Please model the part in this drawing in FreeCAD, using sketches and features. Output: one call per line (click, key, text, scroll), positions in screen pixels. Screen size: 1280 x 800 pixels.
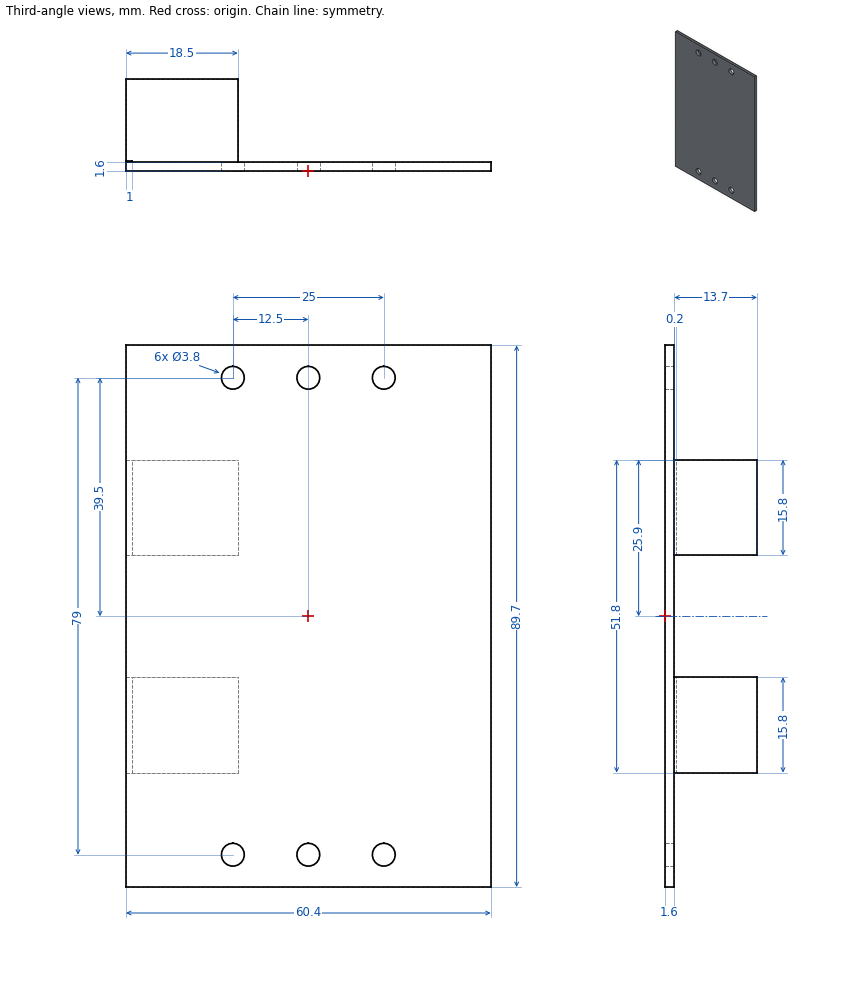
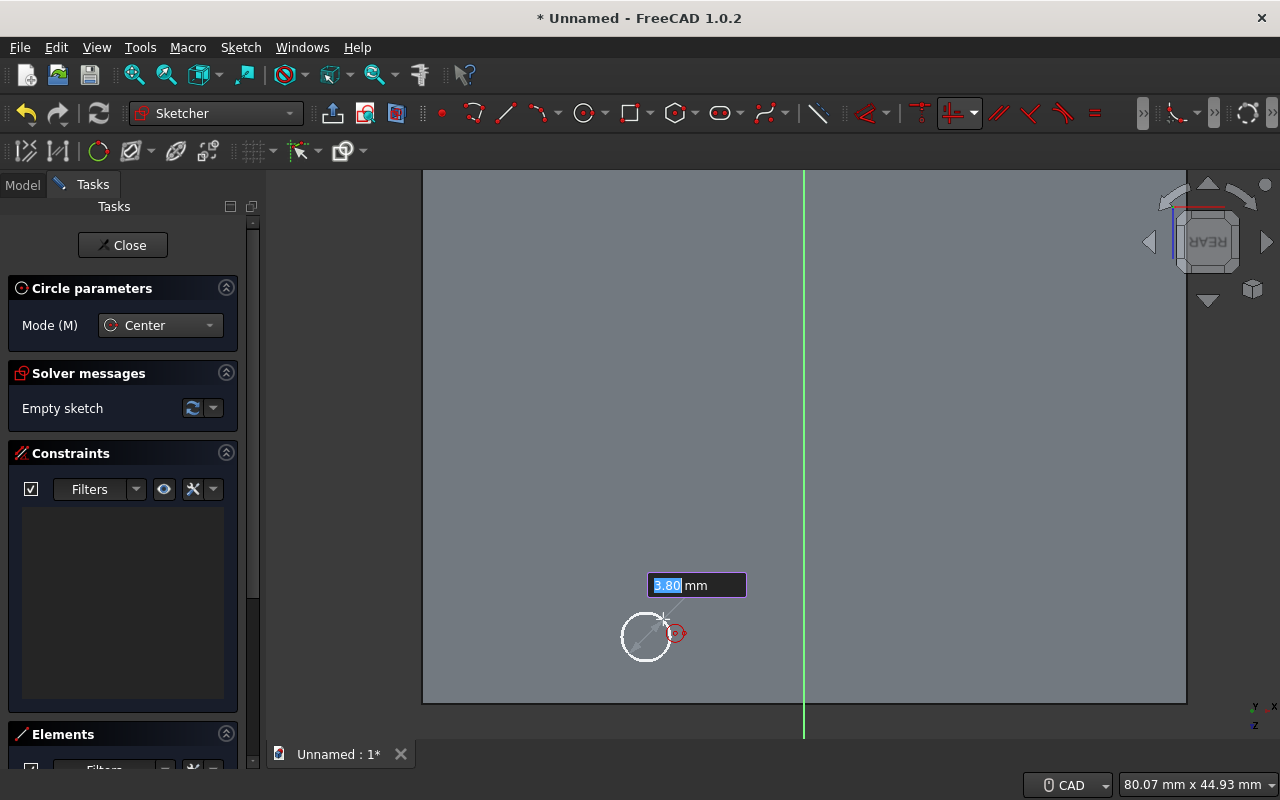
text(3.8)
key(Return)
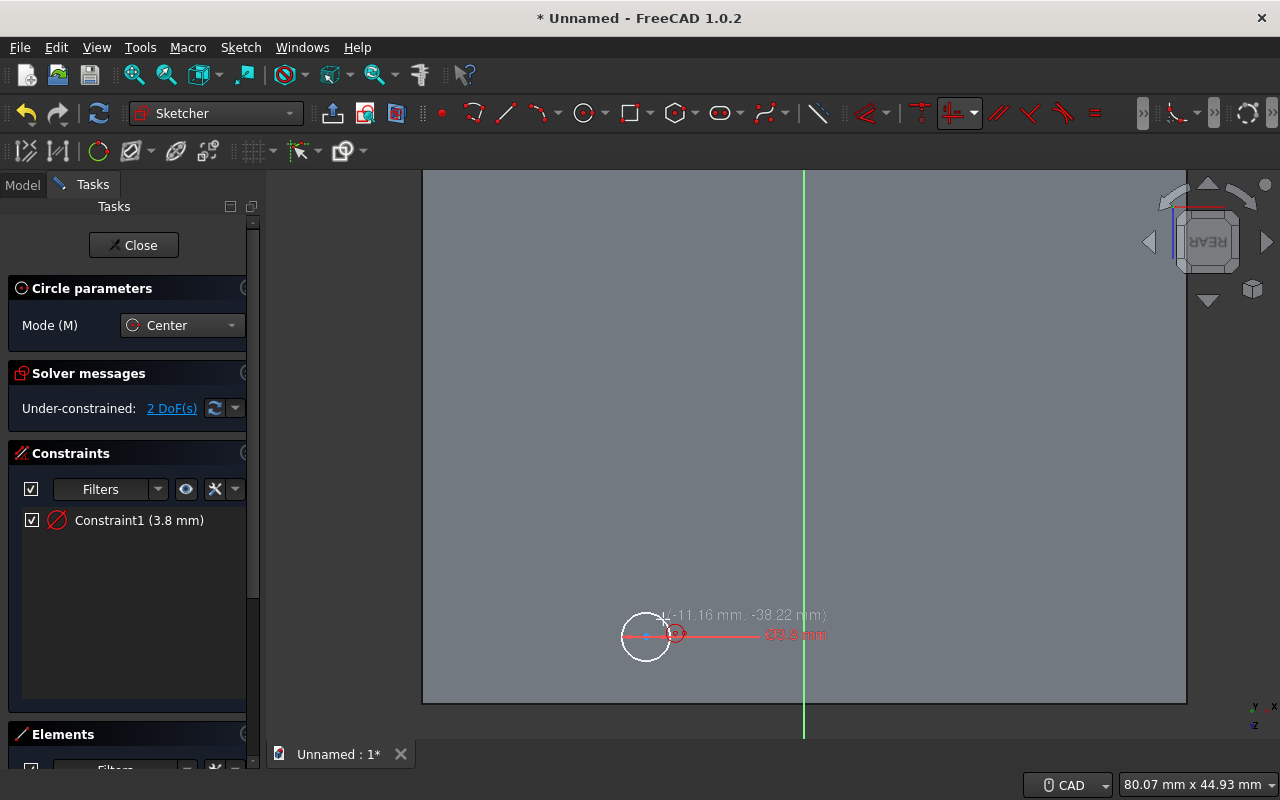
click(963, 636)
move(980, 619)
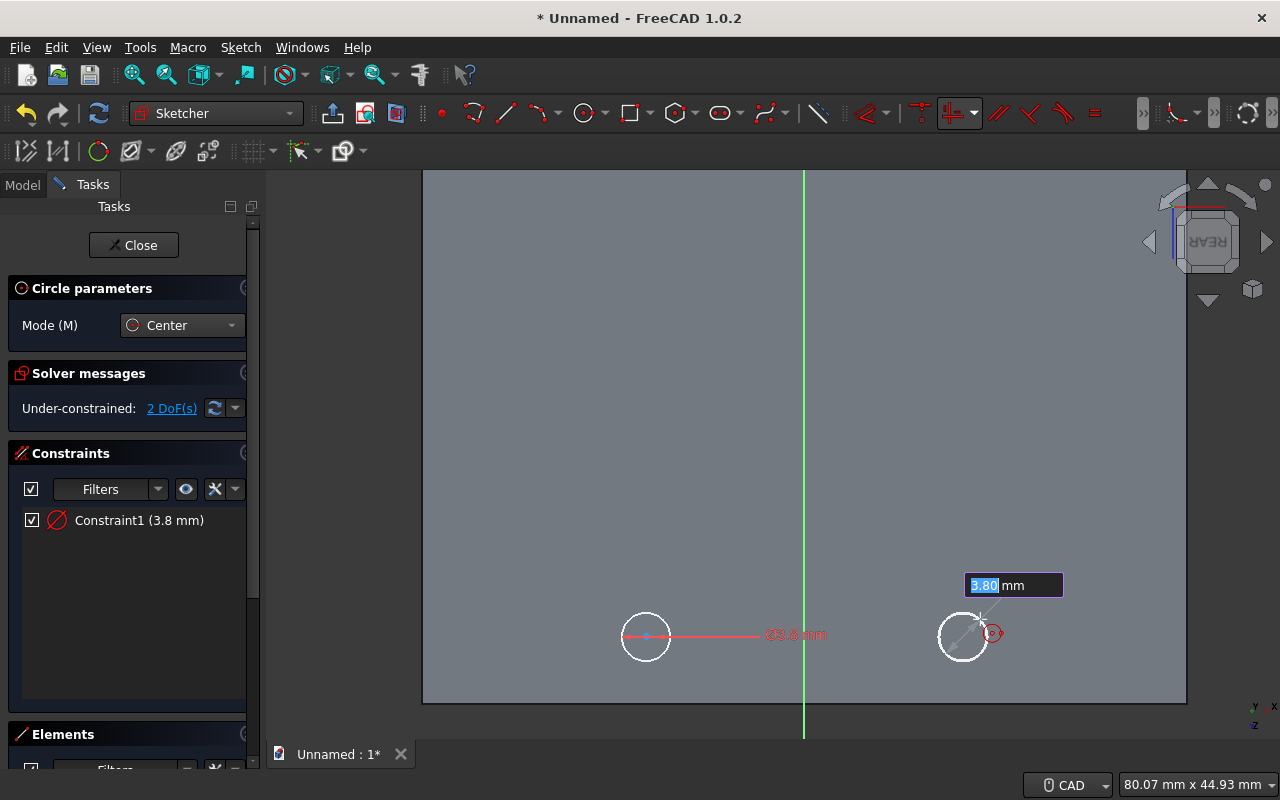
text(3.8)
key(Return)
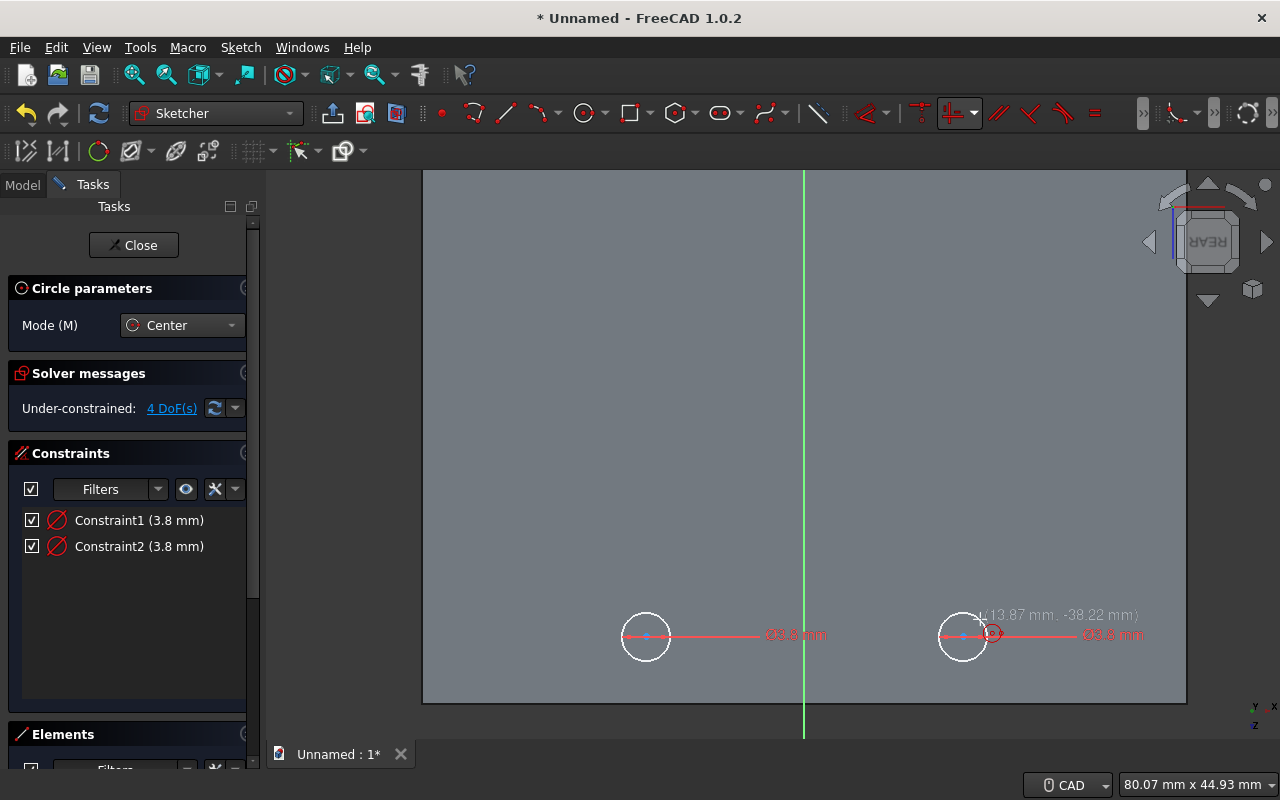
scroll(646, 640, down, 5)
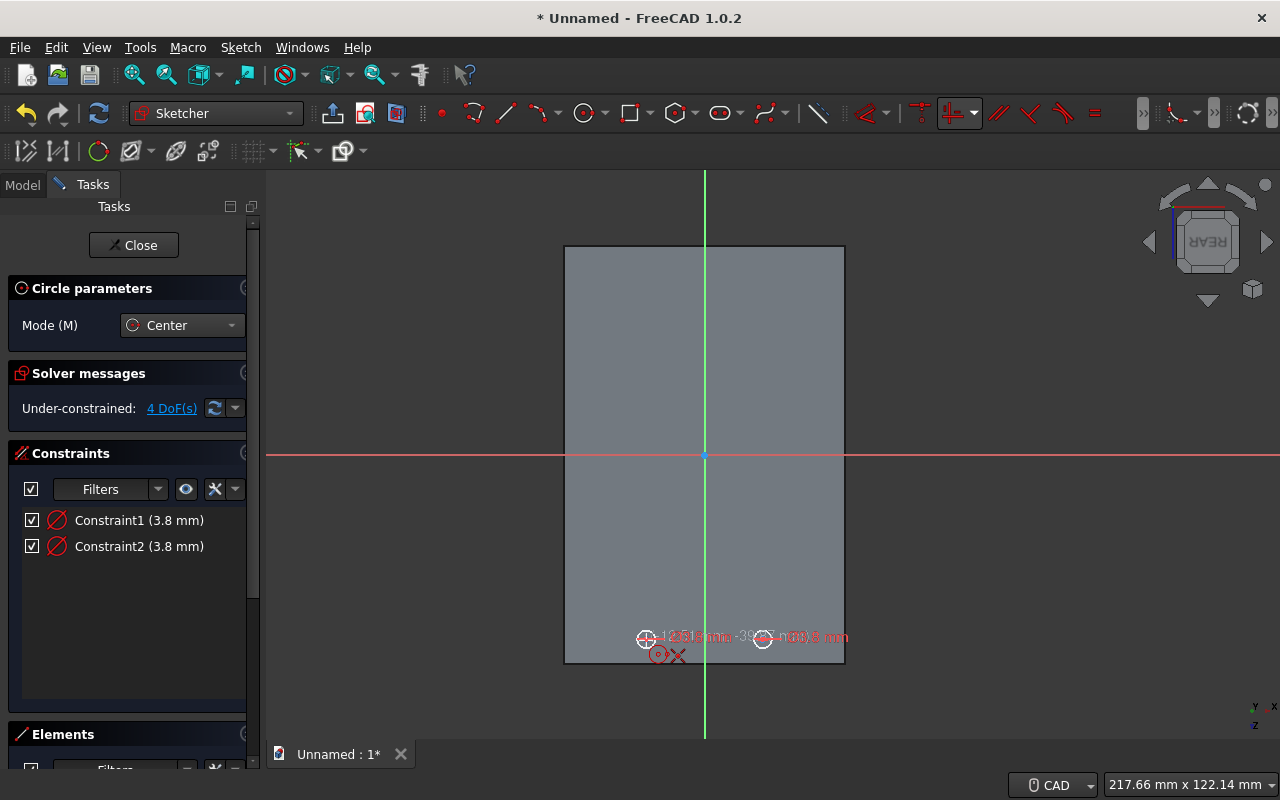
scroll(646, 271, up, 5)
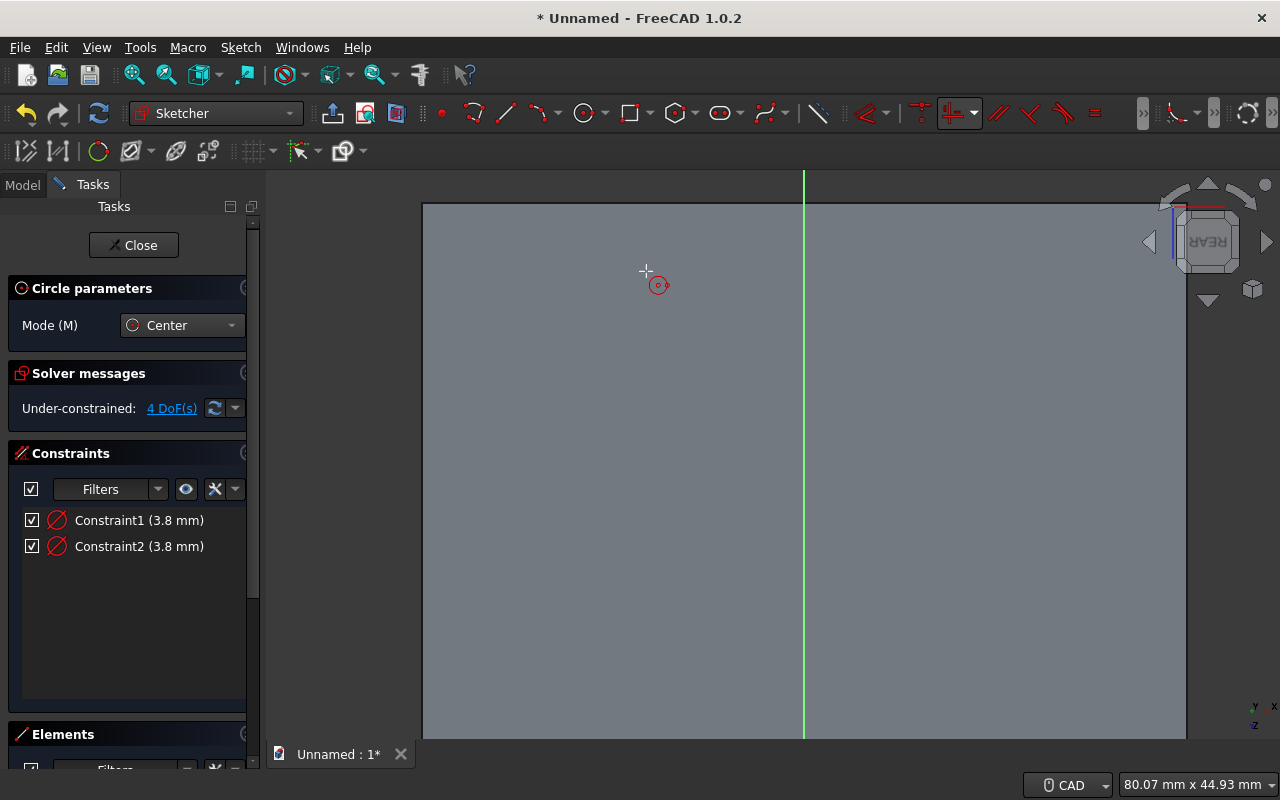
click(646, 271)
move(663, 254)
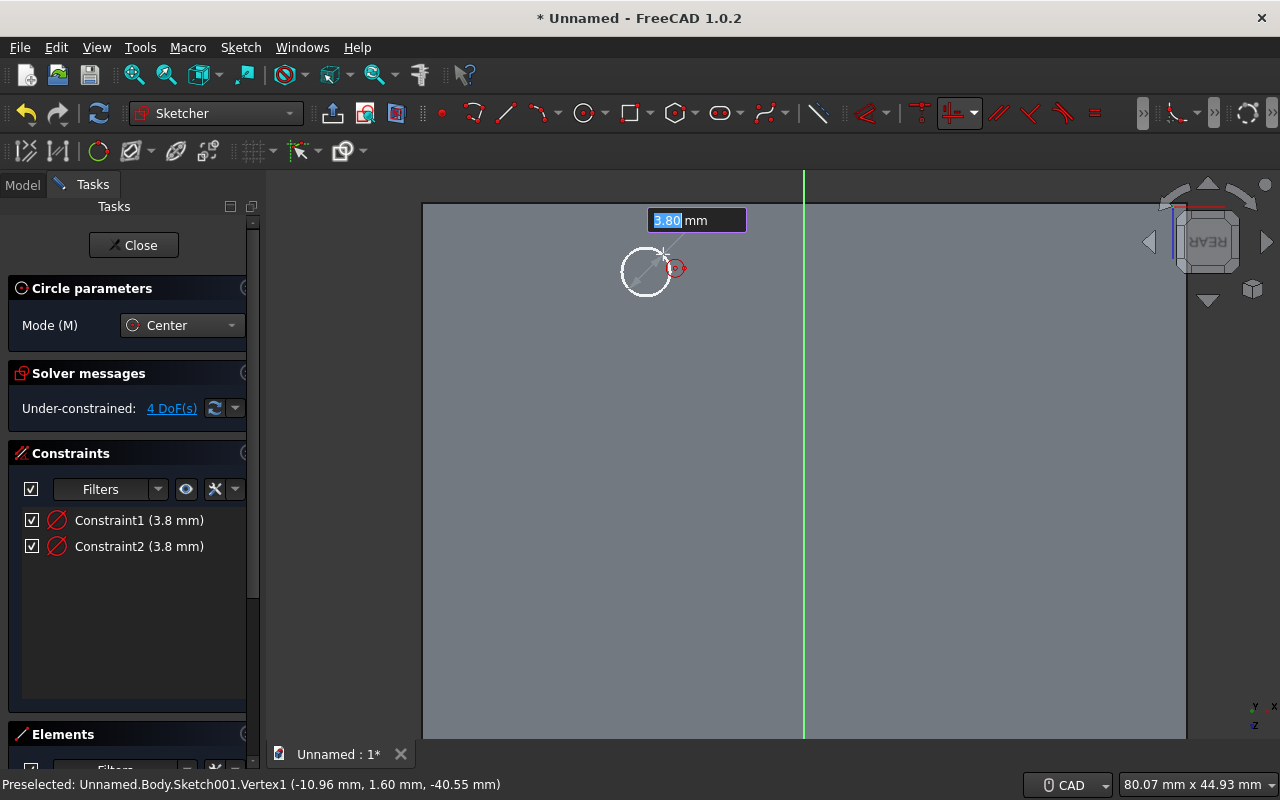
text(3.8)
key(Return)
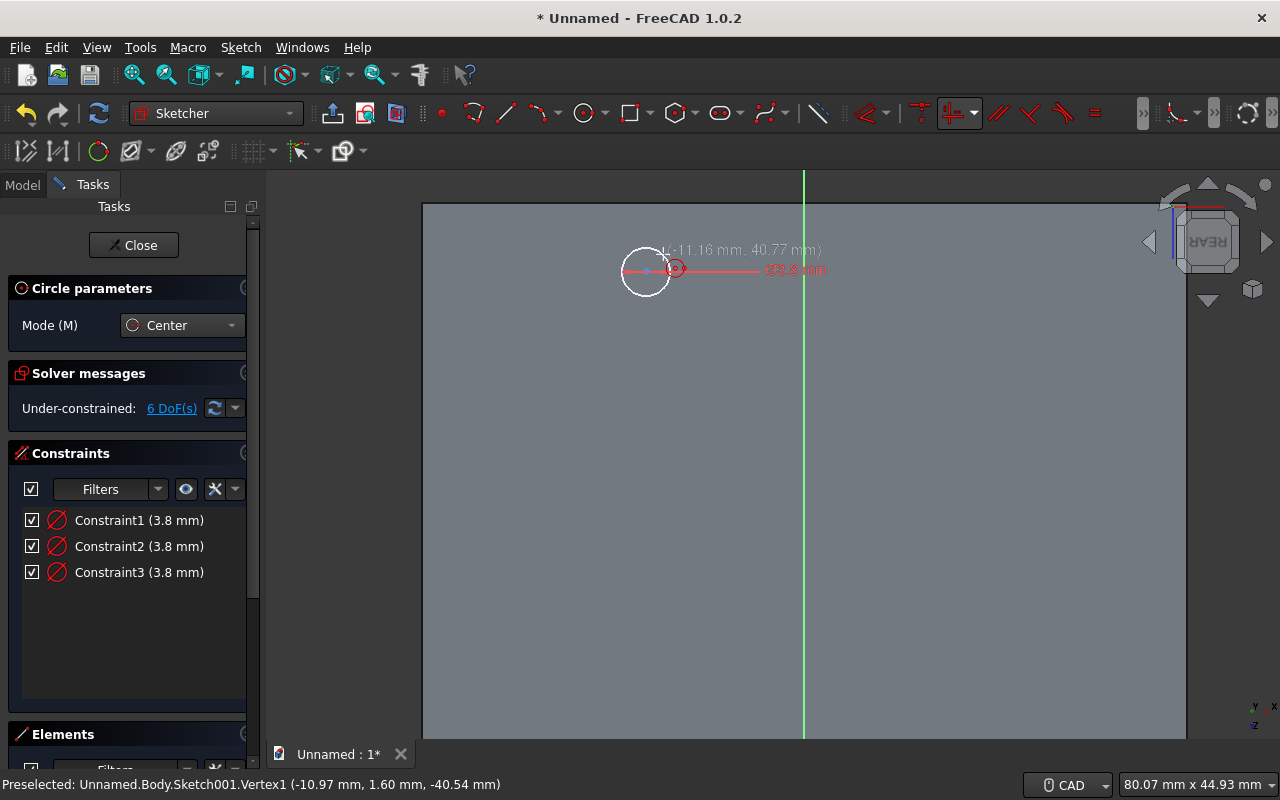
click(963, 271)
move(980, 254)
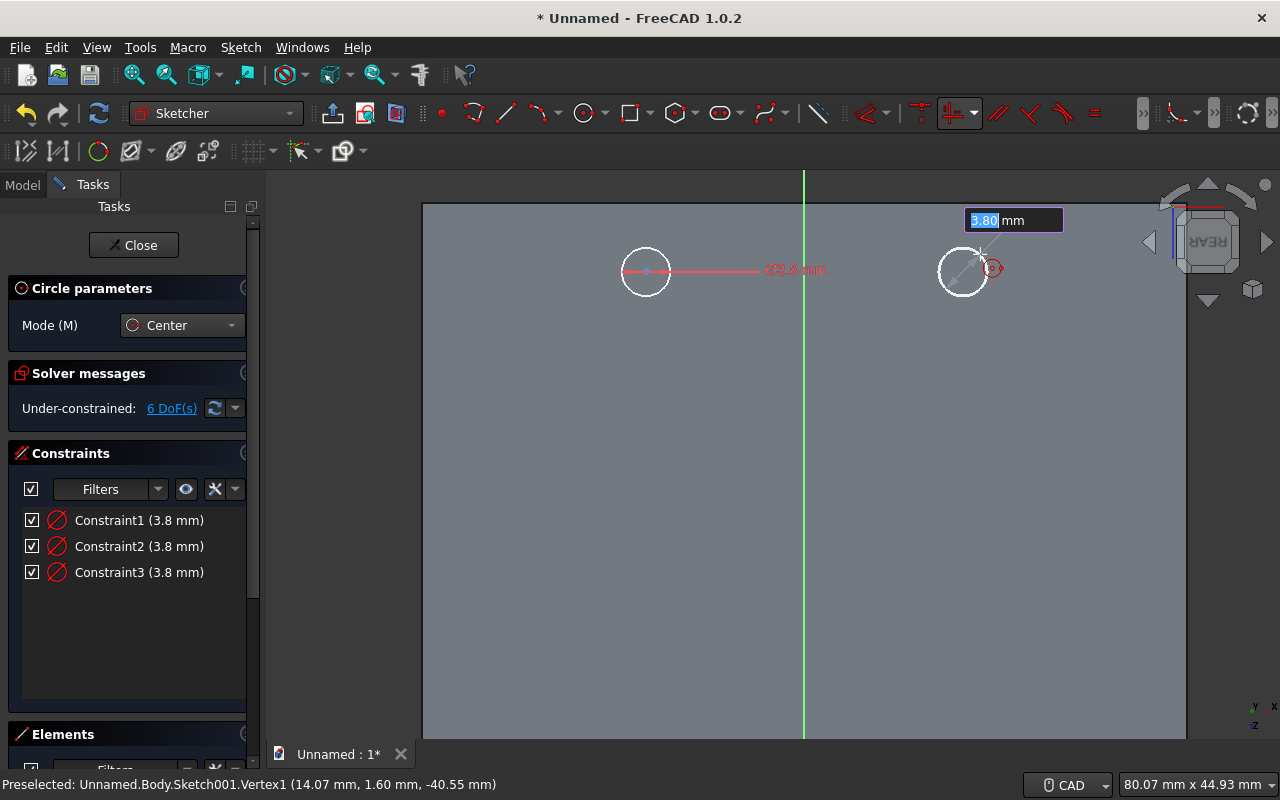
text(3.8)
key(Return)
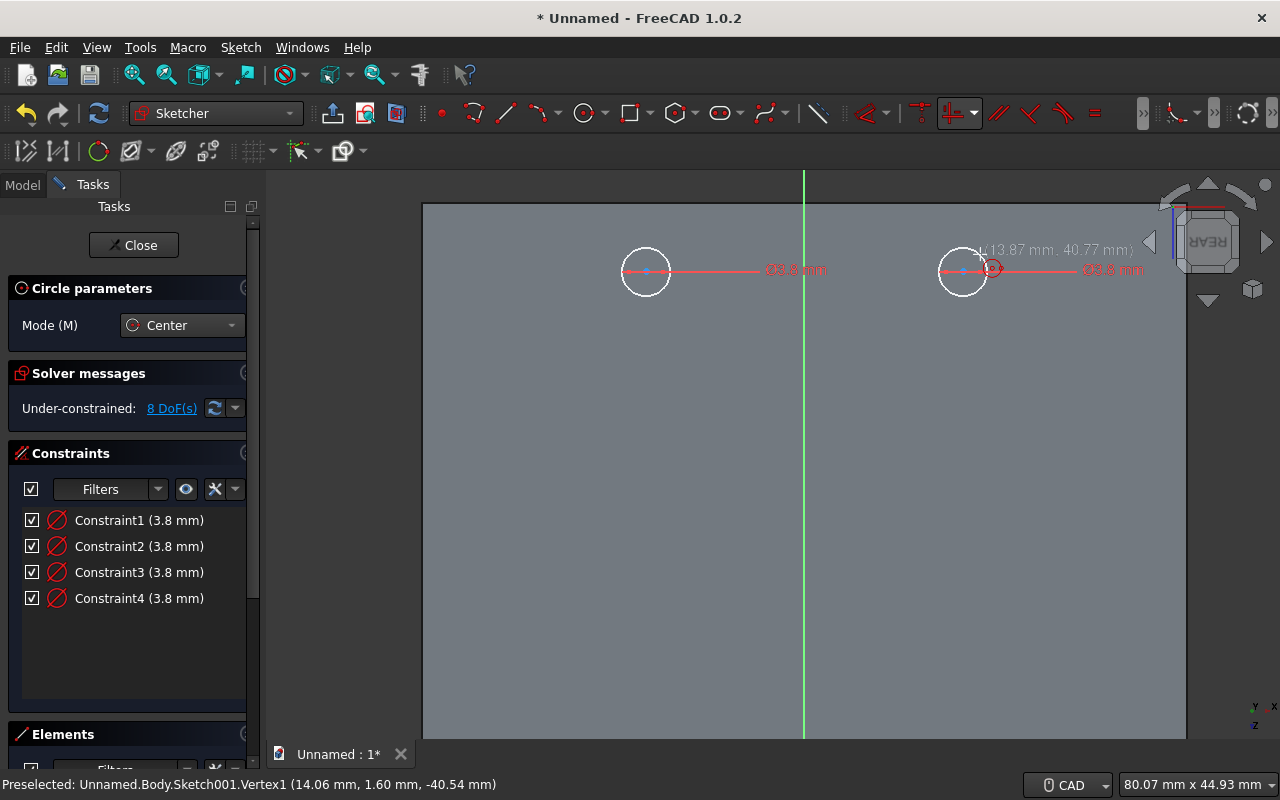
click(804, 271)
move(821, 254)